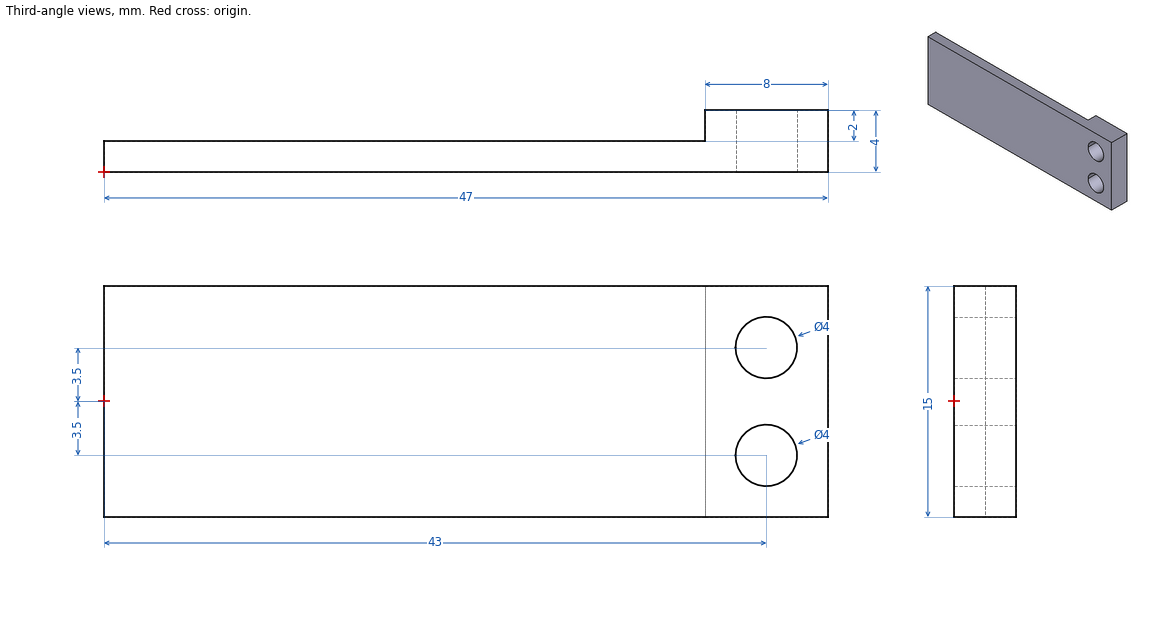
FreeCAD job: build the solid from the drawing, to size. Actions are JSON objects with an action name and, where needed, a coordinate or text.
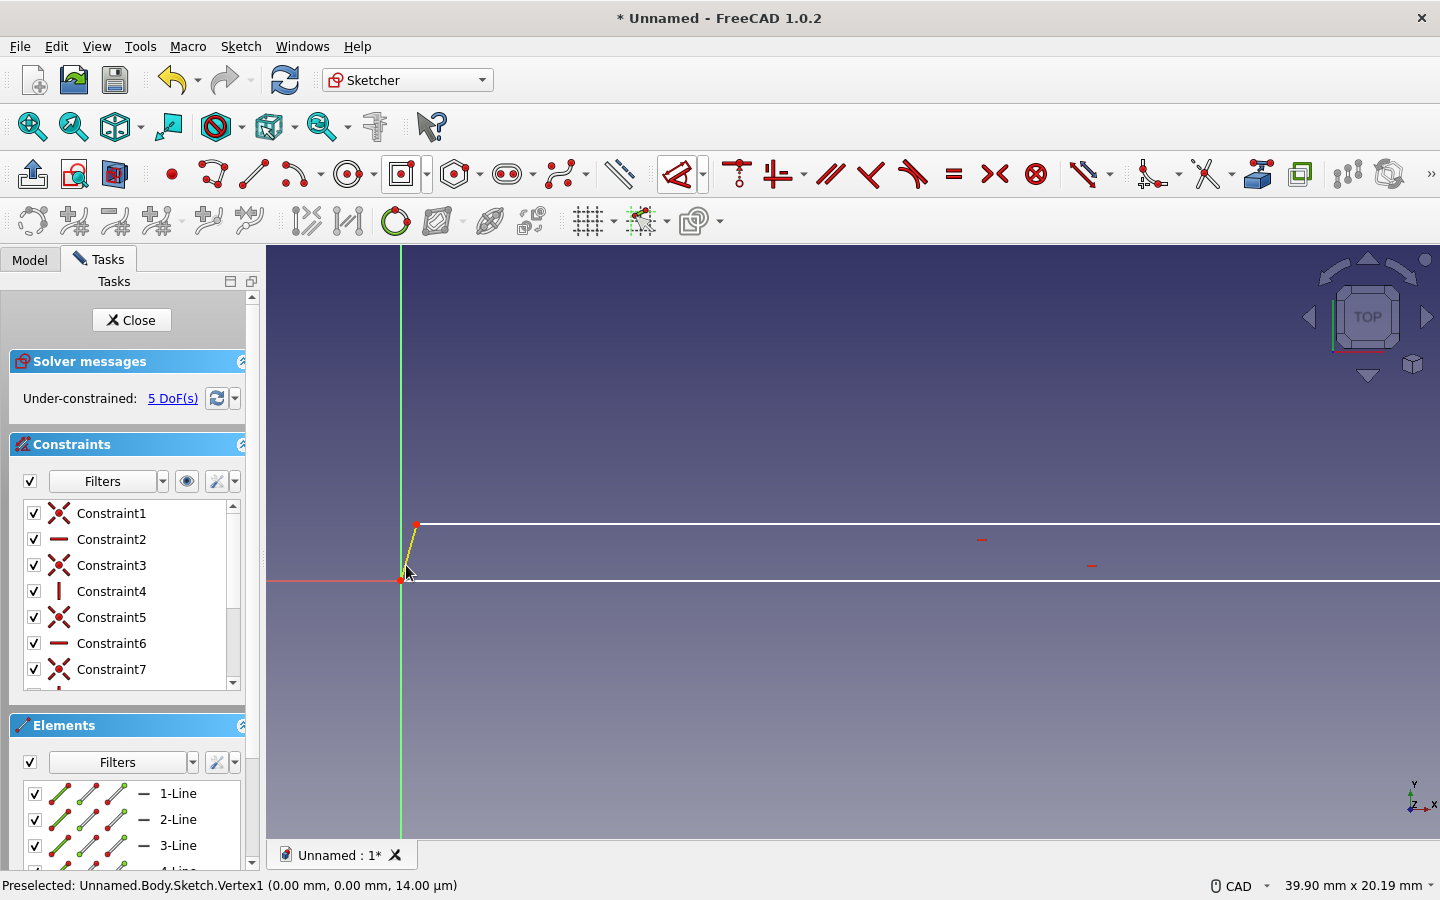
{"action": "left_click", "coordinate": [406, 564]}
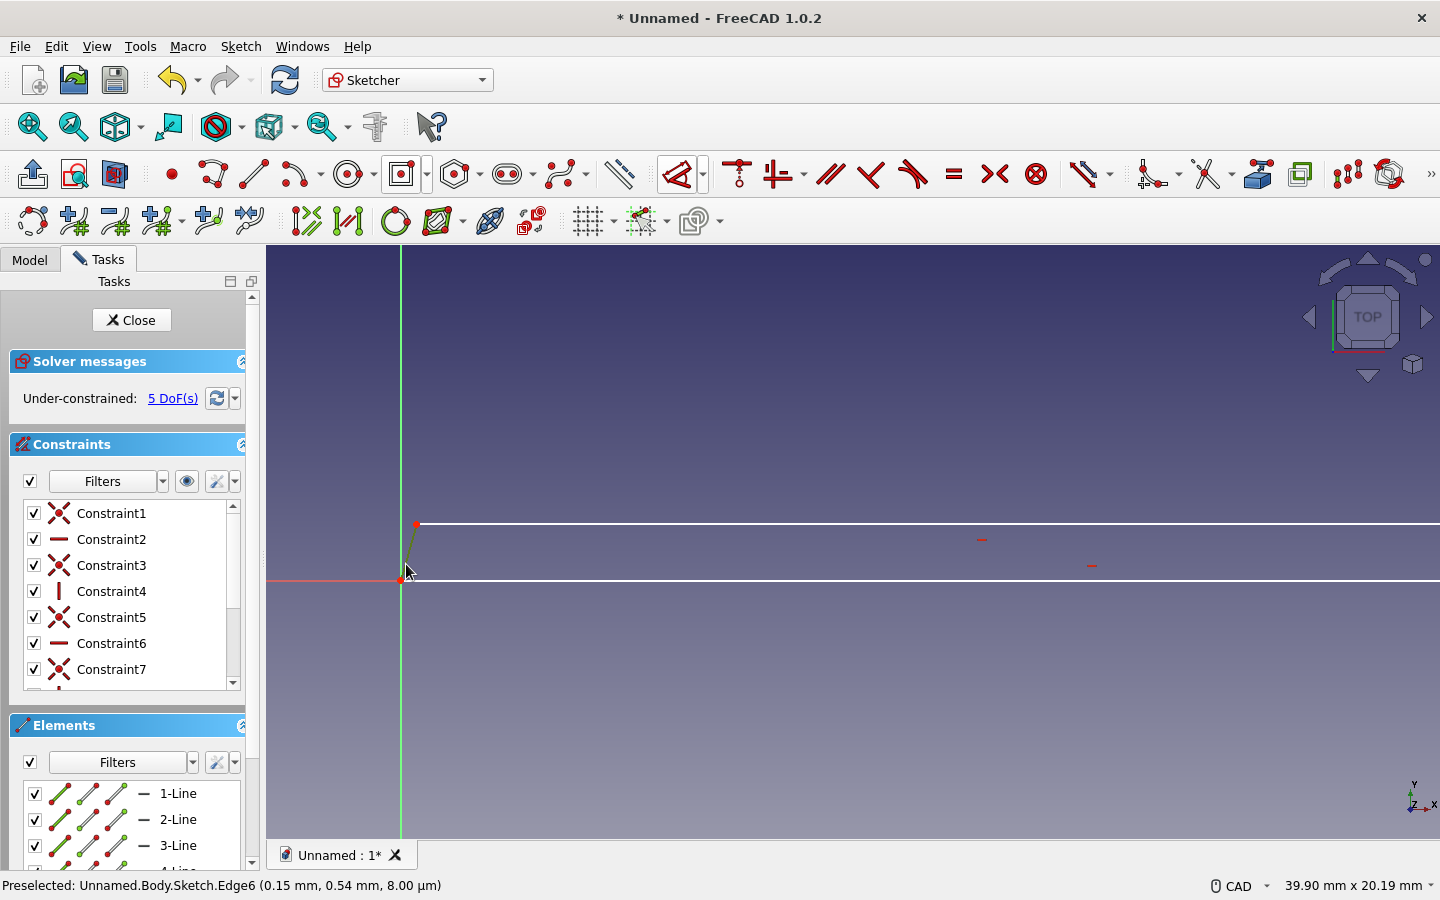
{"action": "left_click", "coordinate": [804, 174]}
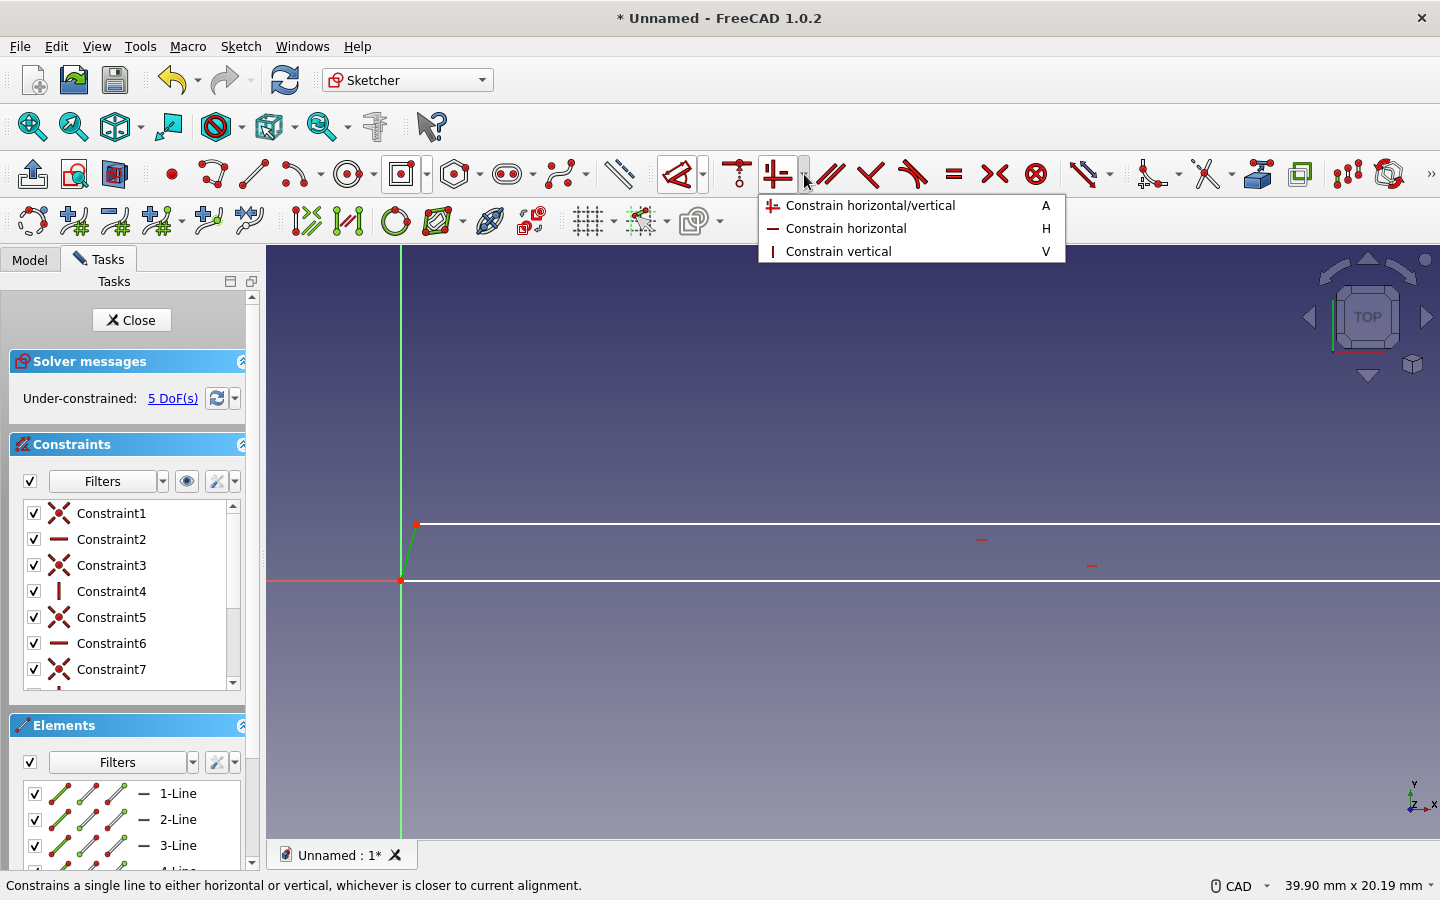
{"action": "left_click", "coordinate": [912, 252]}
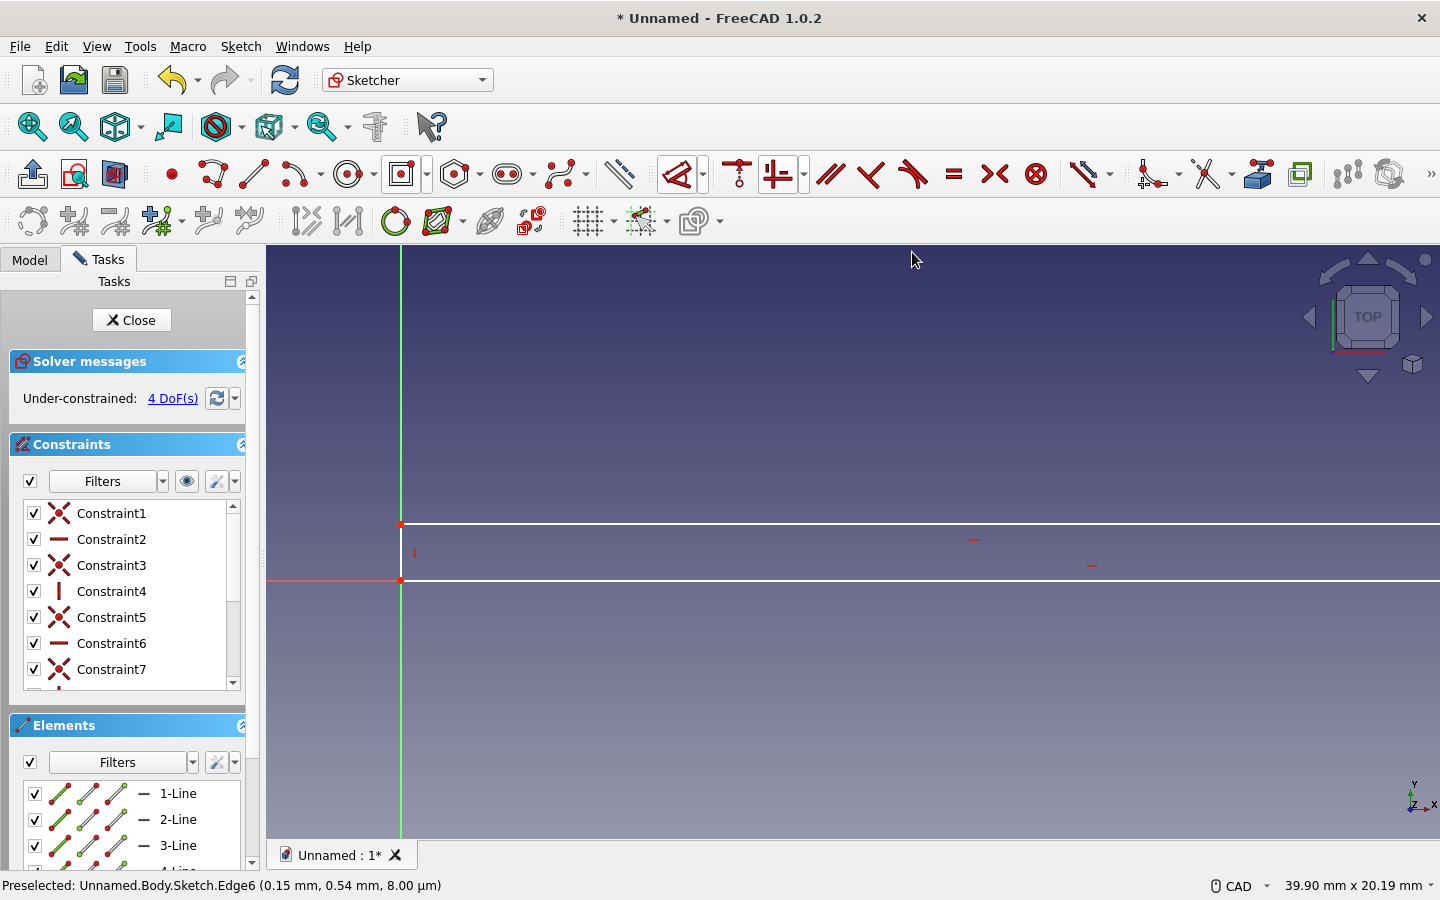
{"action": "scroll", "coordinate": [410, 567], "scroll_direction": "down", "scroll_amount": 3}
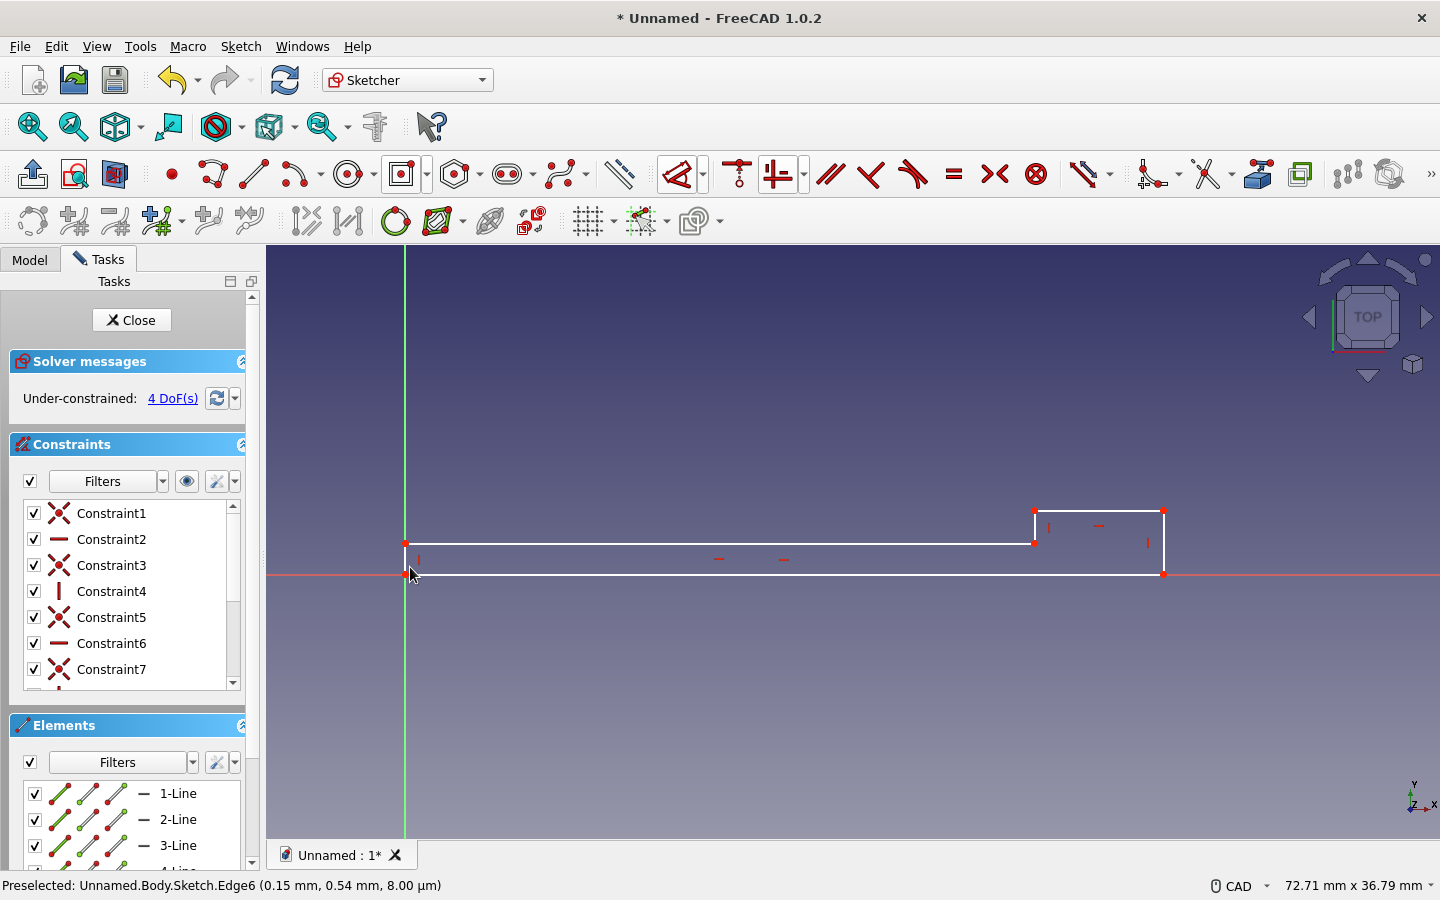
{"action": "left_click", "coordinate": [1164, 556]}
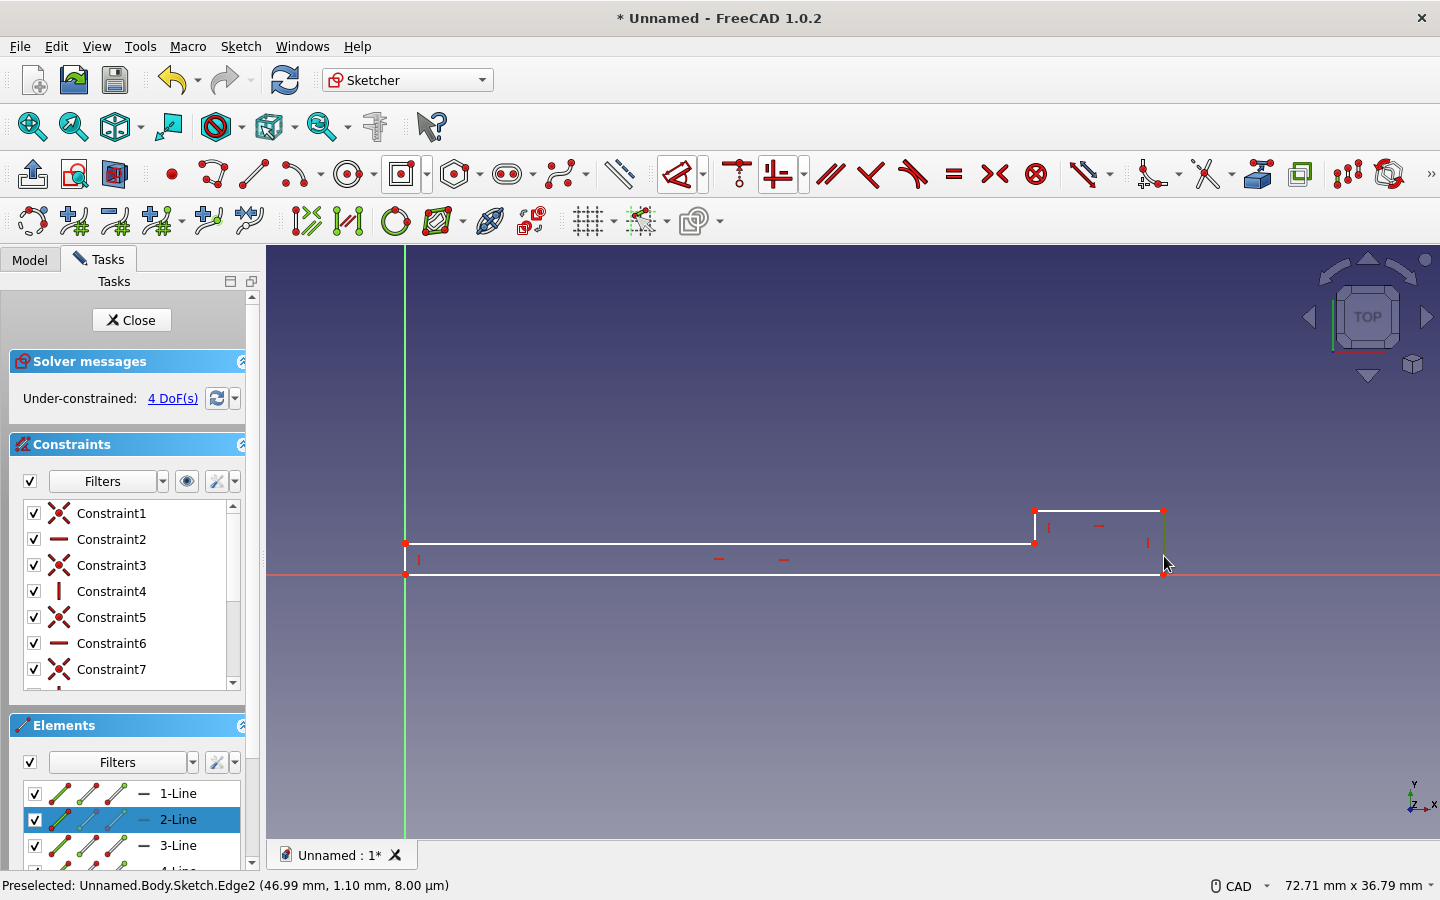
{"action": "key", "text": "i"}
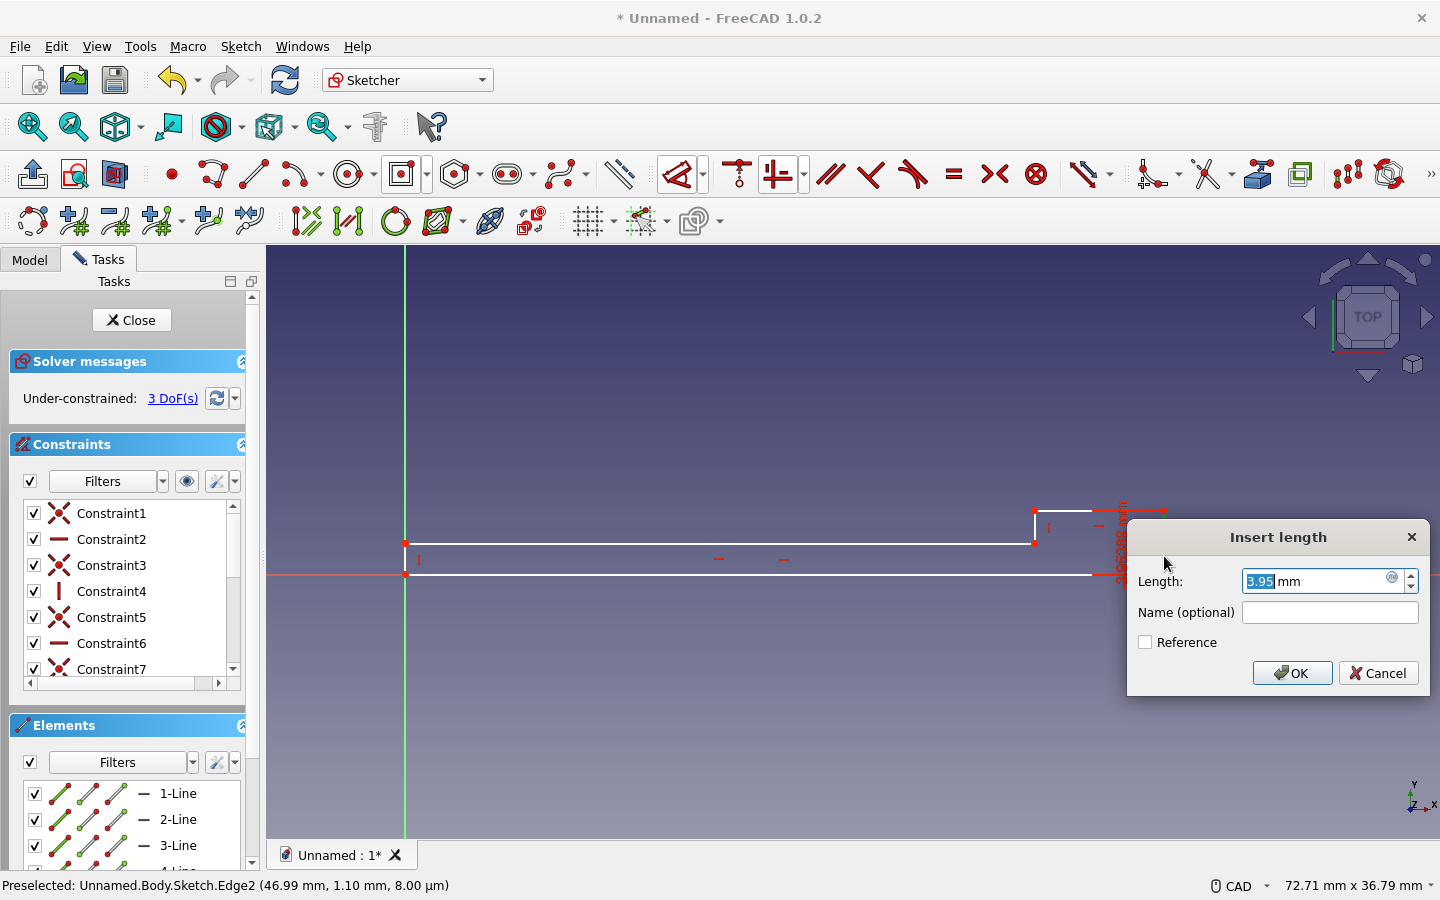
{"action": "type", "text": "4"}
{"action": "key", "text": "Return"}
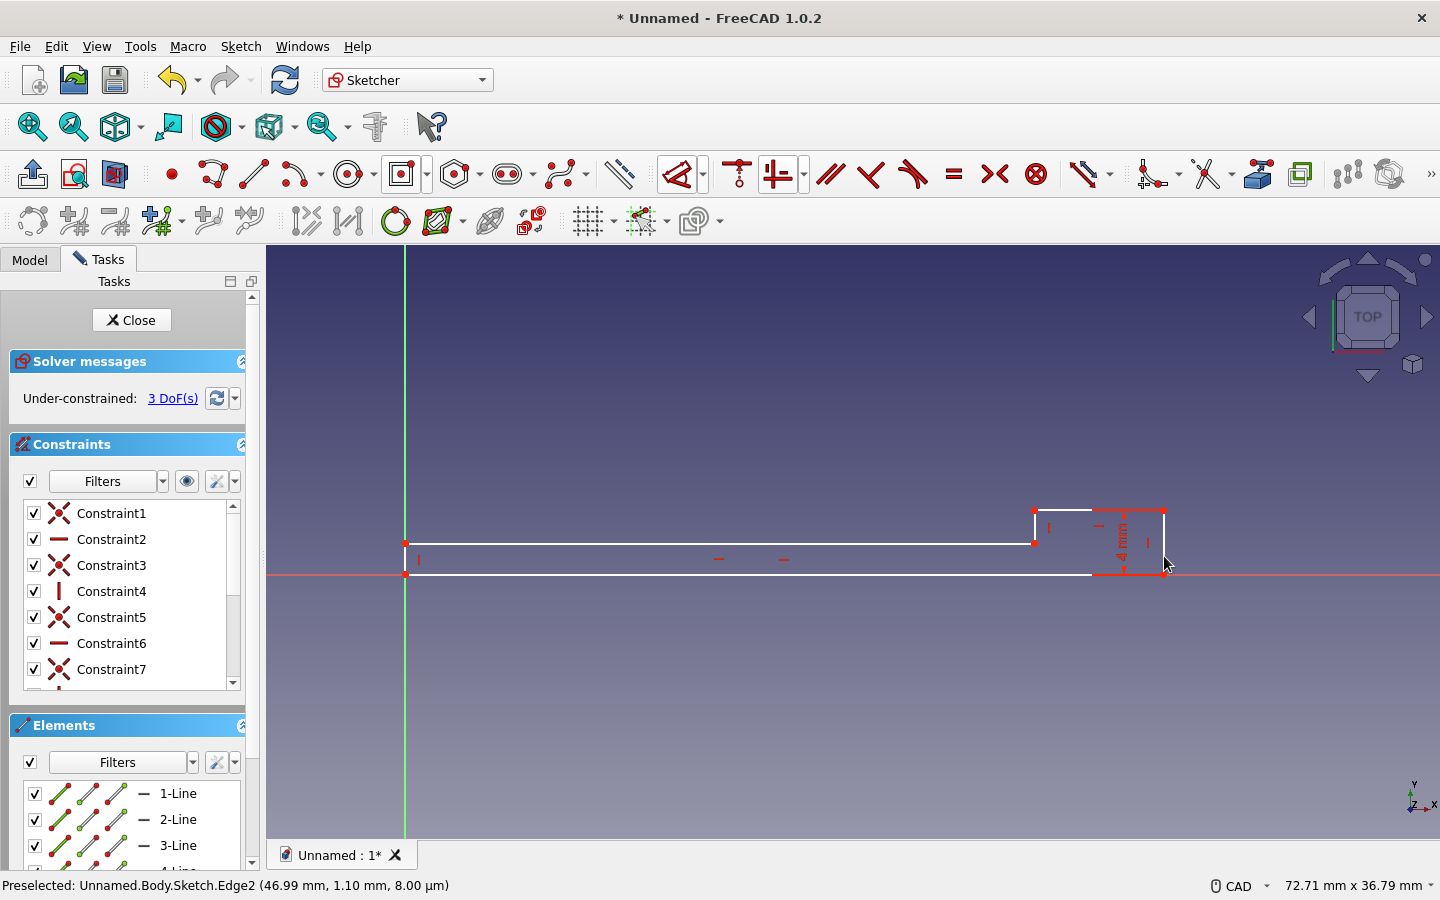
{"action": "left_click", "coordinate": [1125, 510]}